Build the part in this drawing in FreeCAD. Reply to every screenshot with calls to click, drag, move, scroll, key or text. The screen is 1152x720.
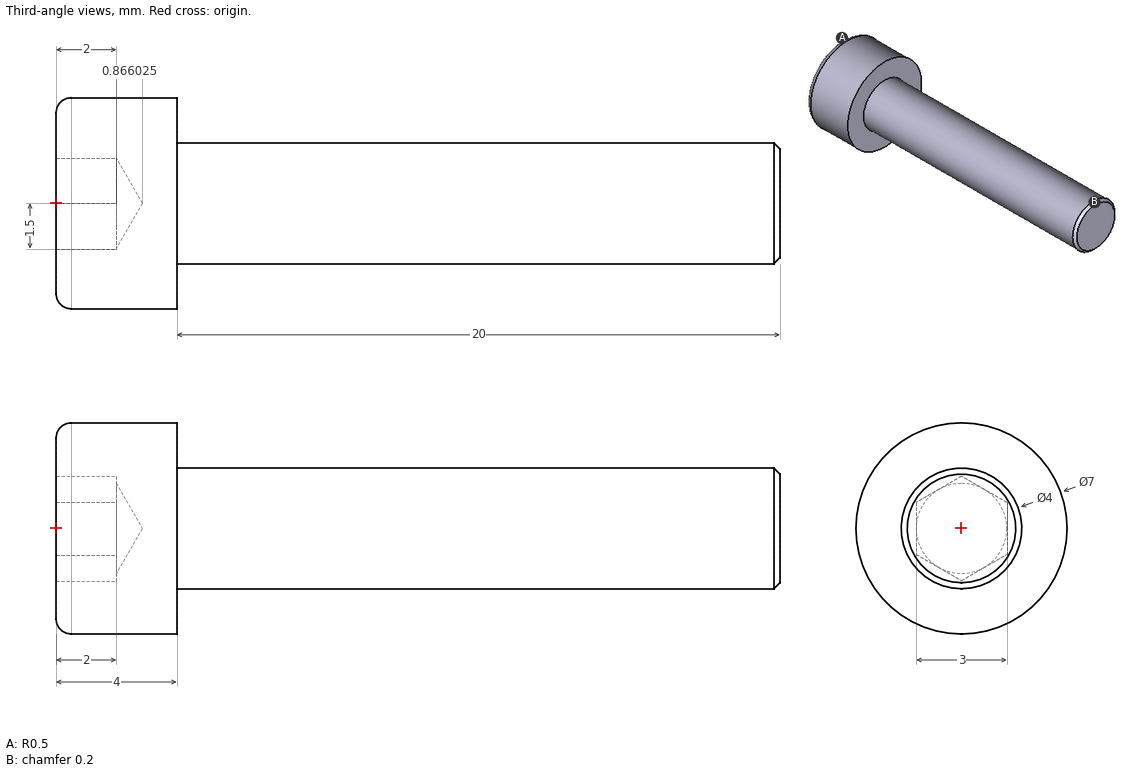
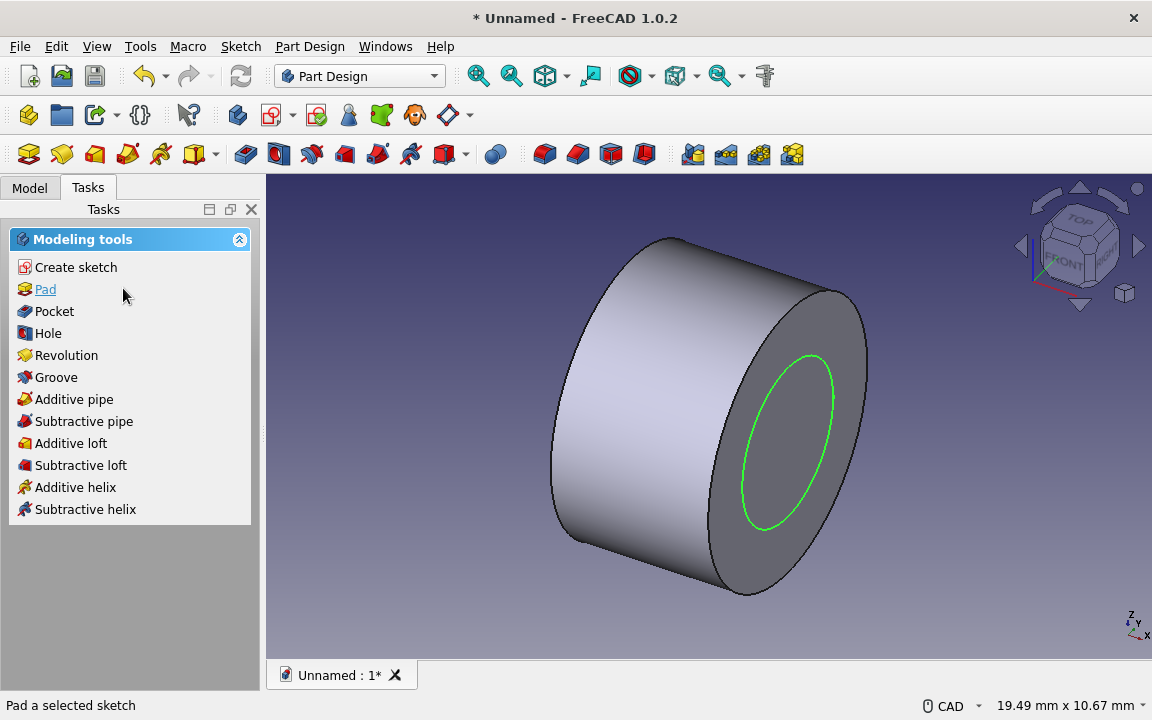
click(29, 154)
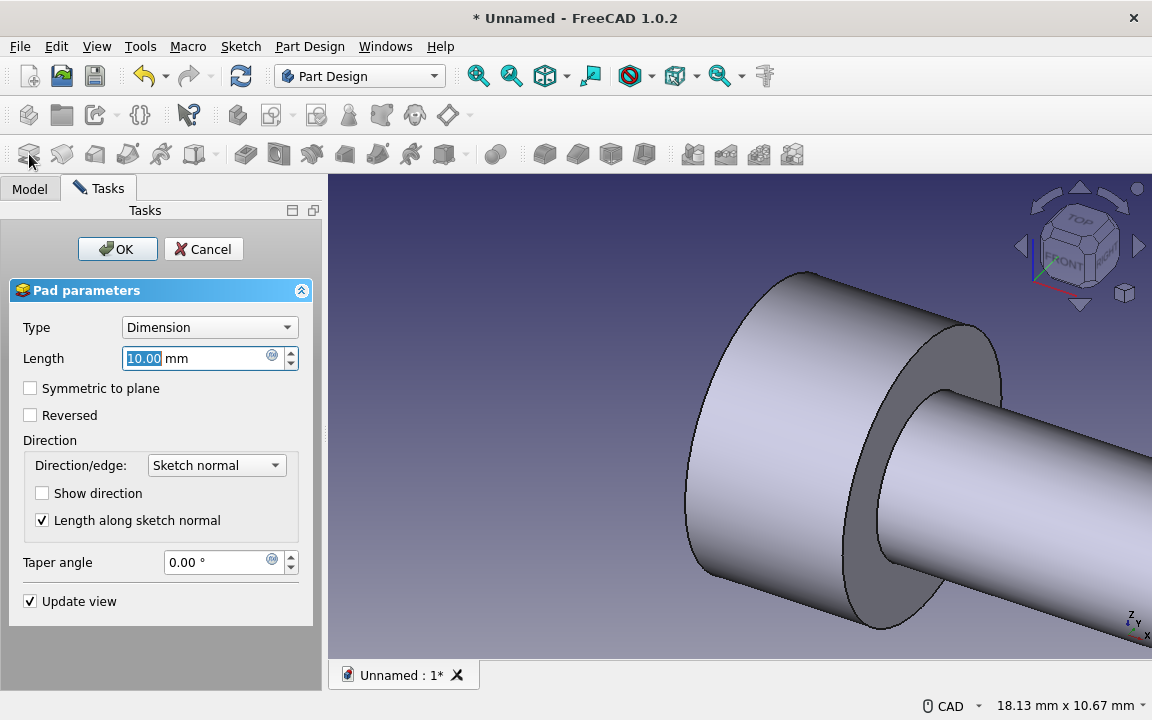
text(20)
key(Tab)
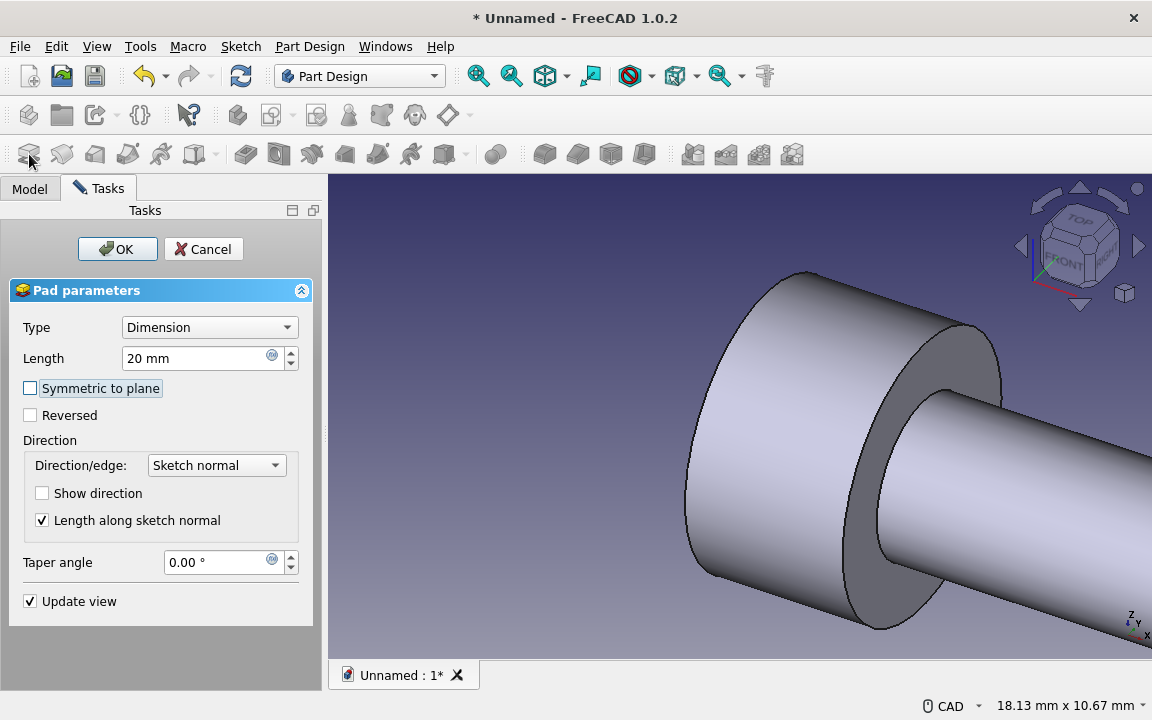
click(118, 249)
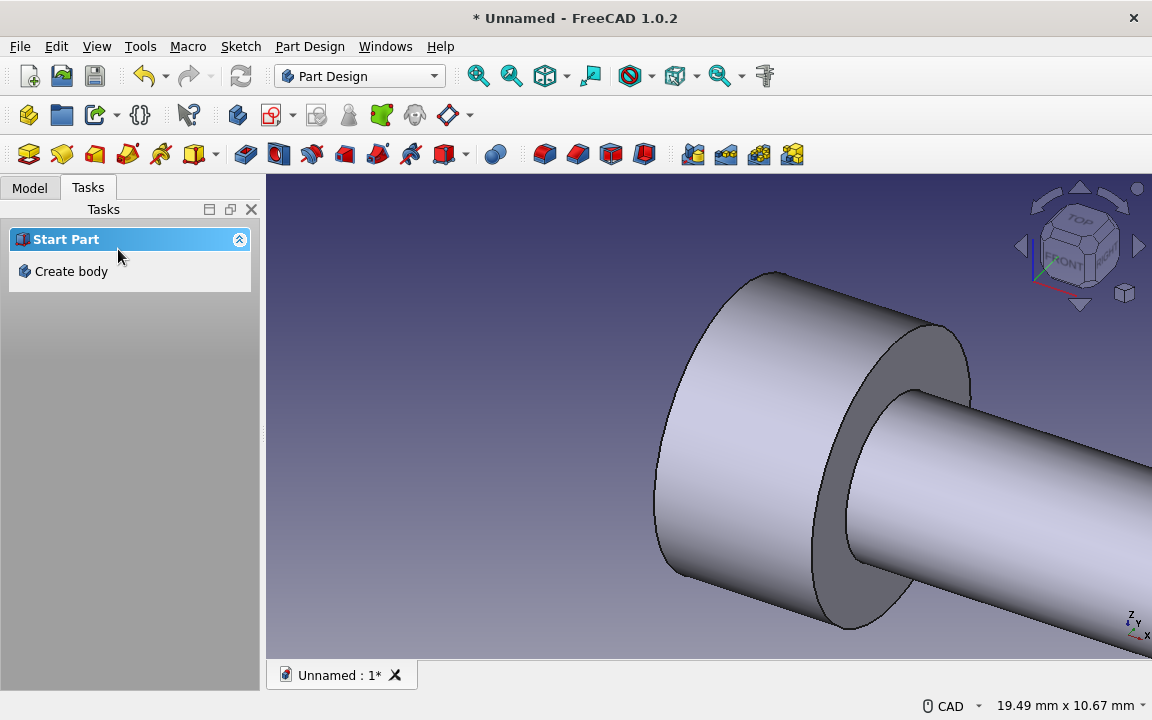
click(479, 76)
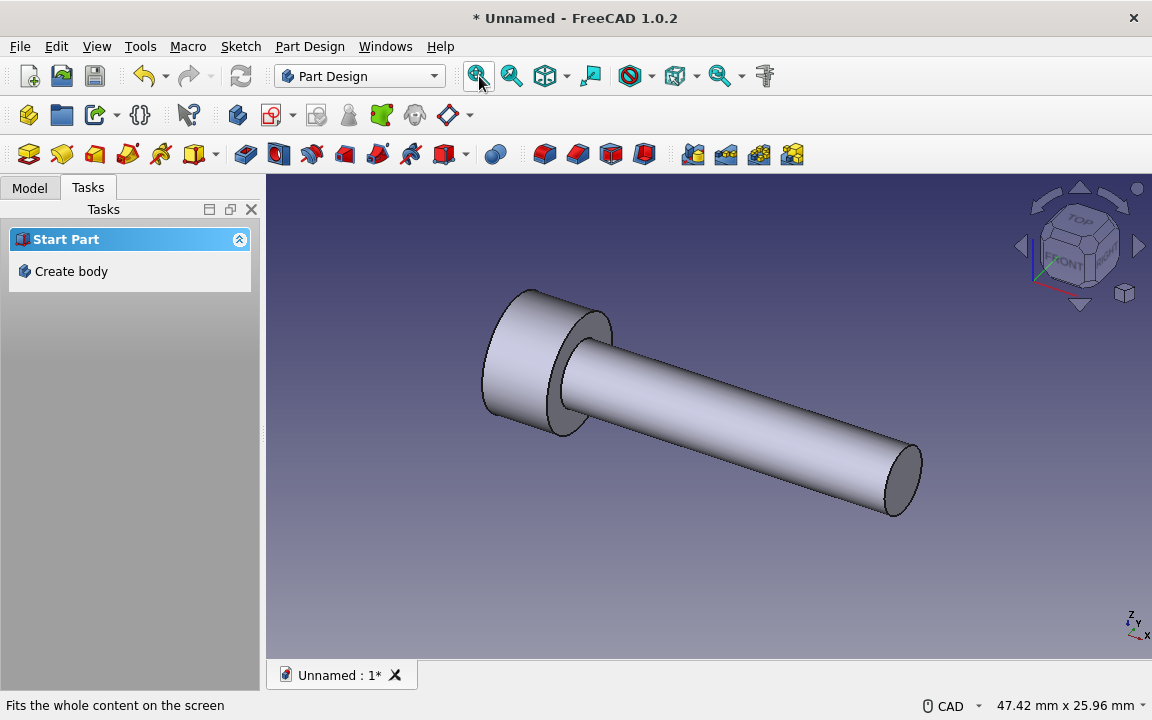
key(6)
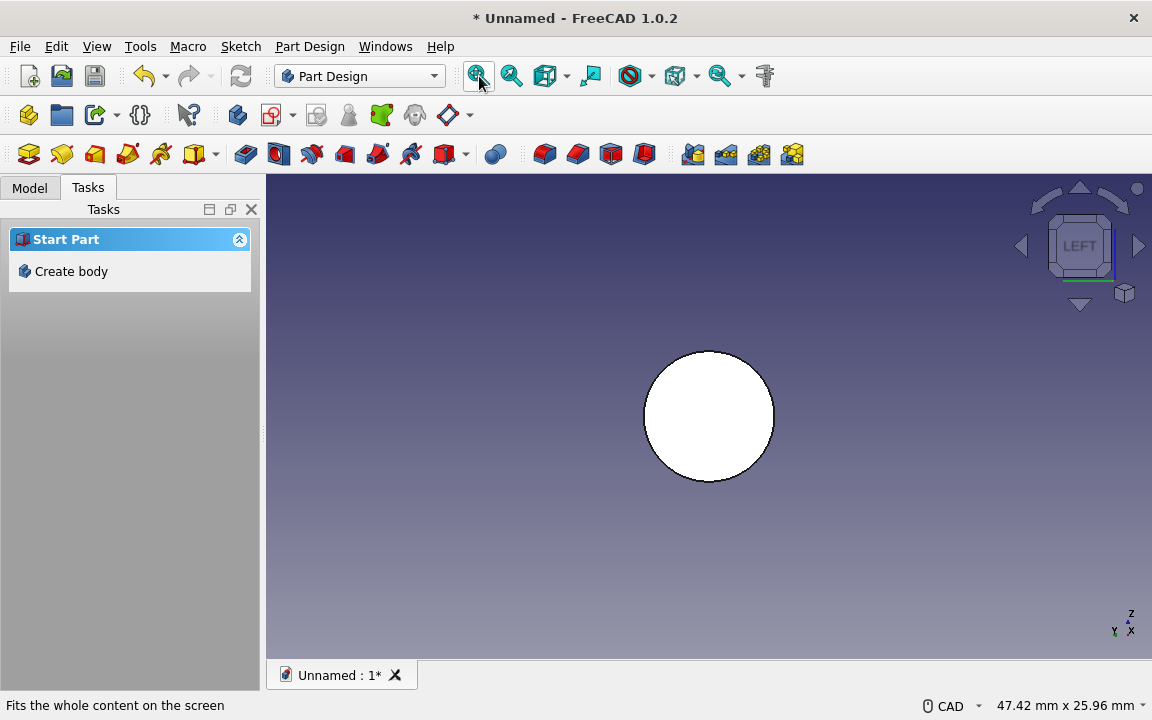
click(479, 76)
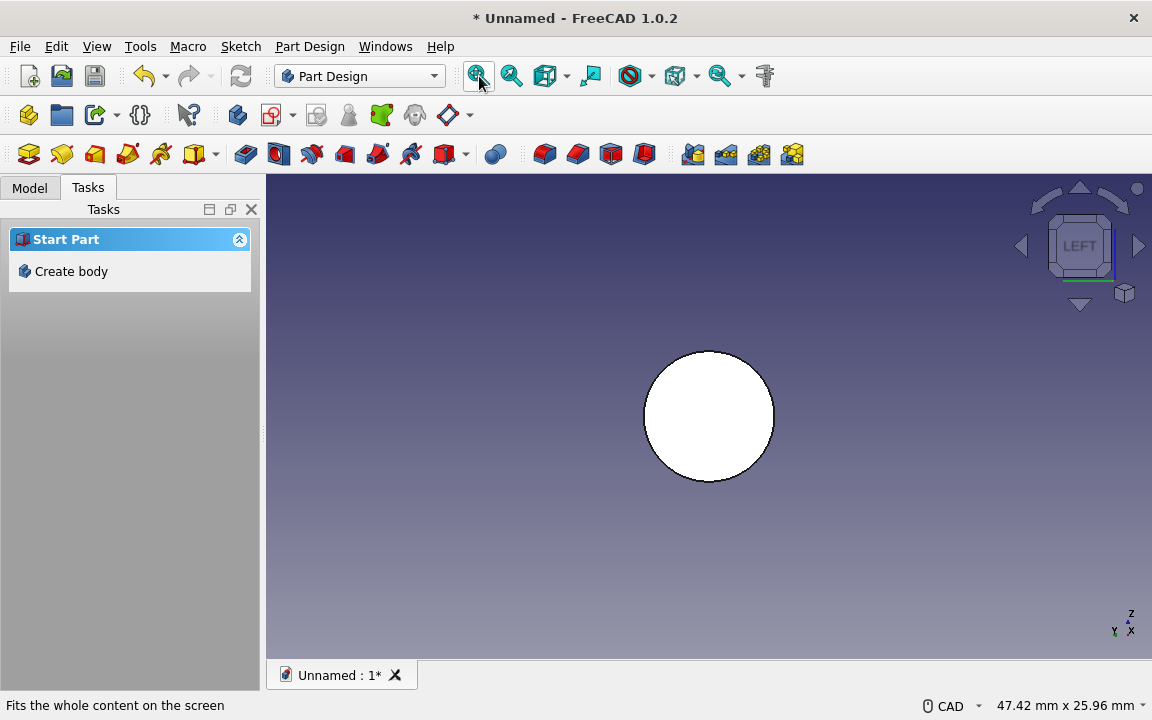
click(709, 415)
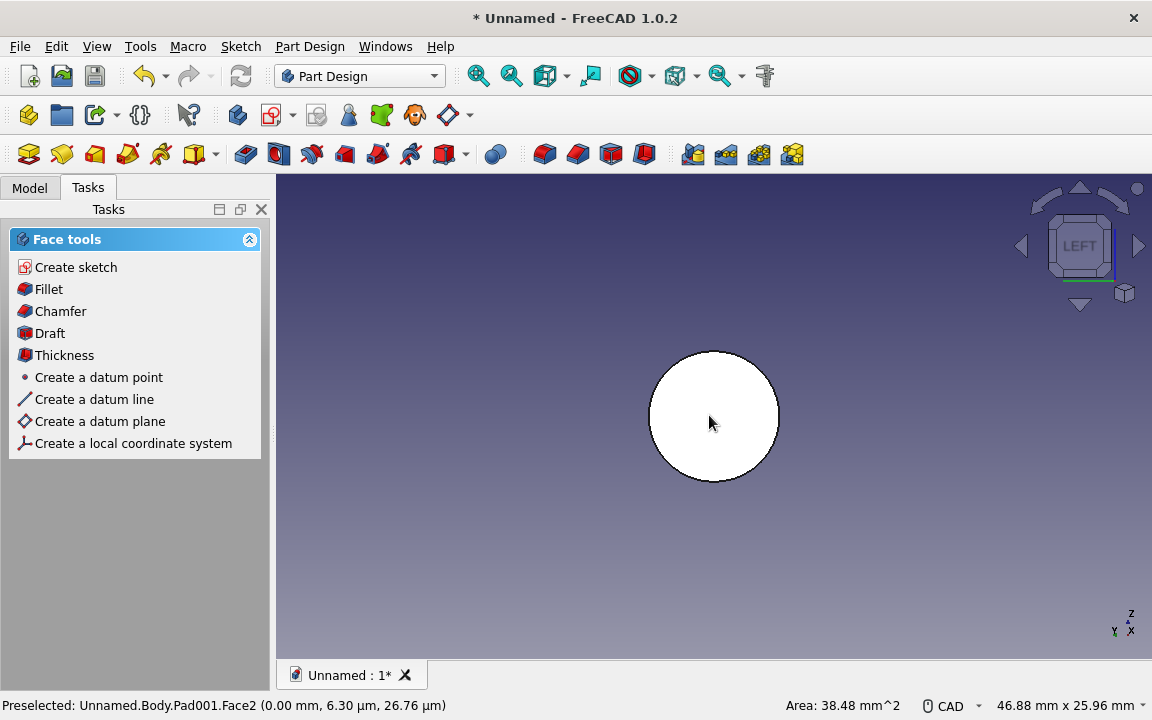
click(270, 116)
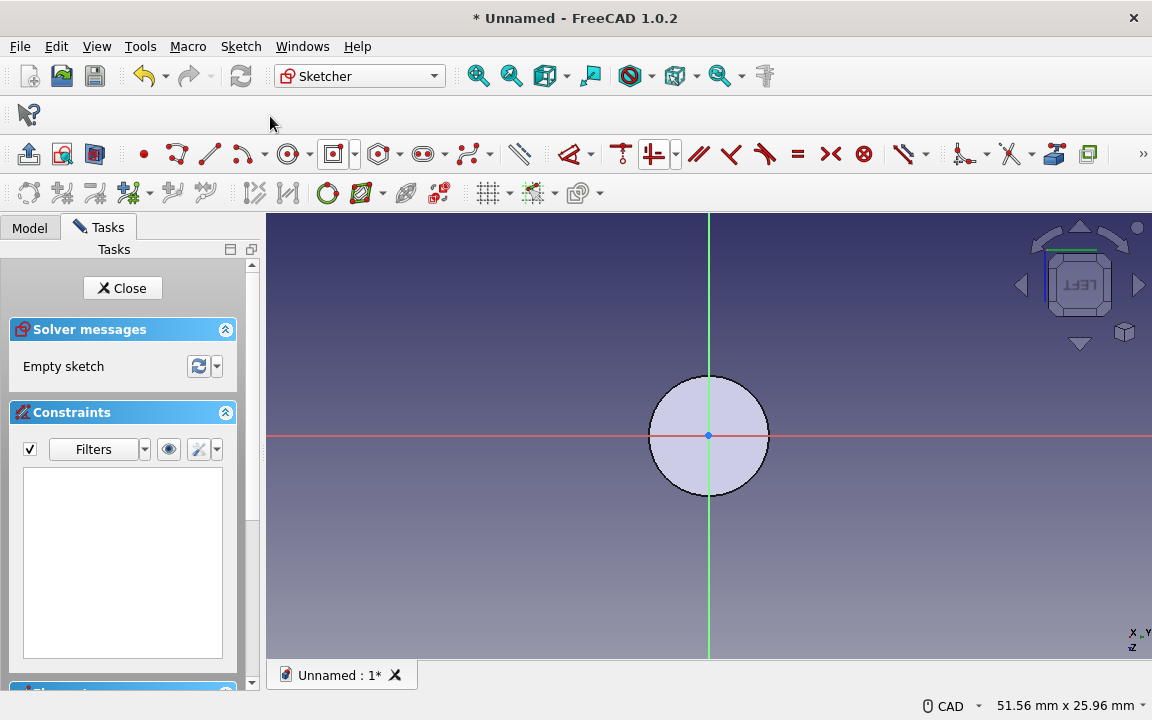
scroll(726, 436, up, 8)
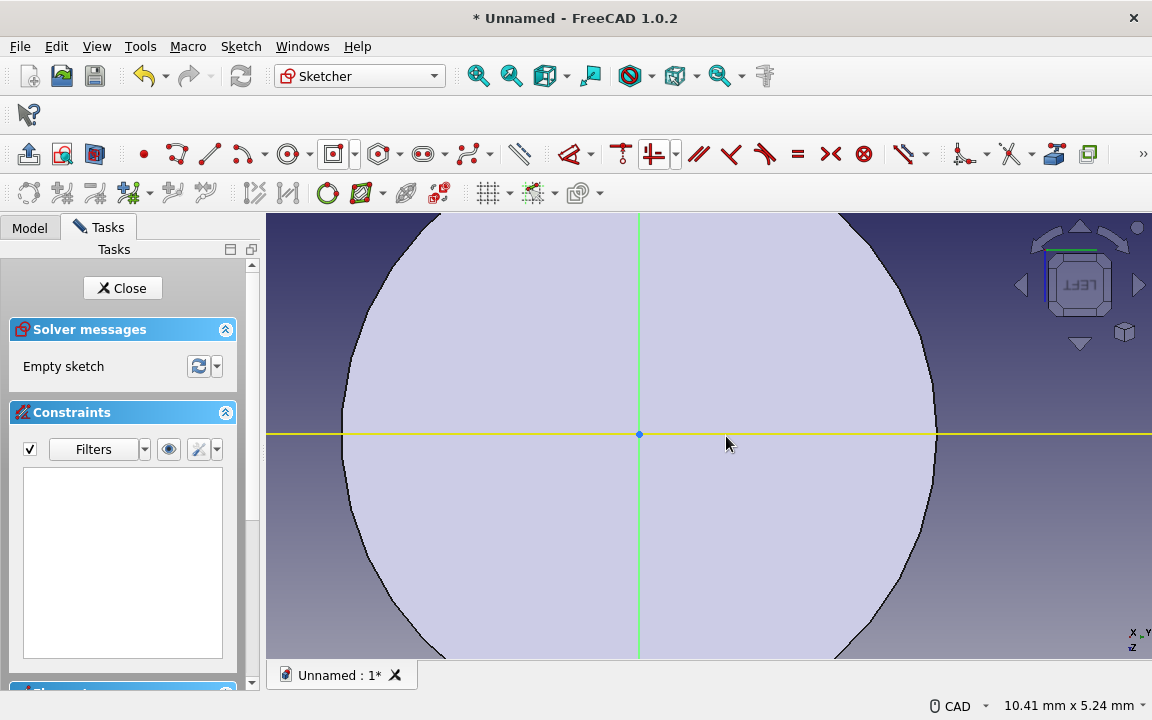
click(378, 154)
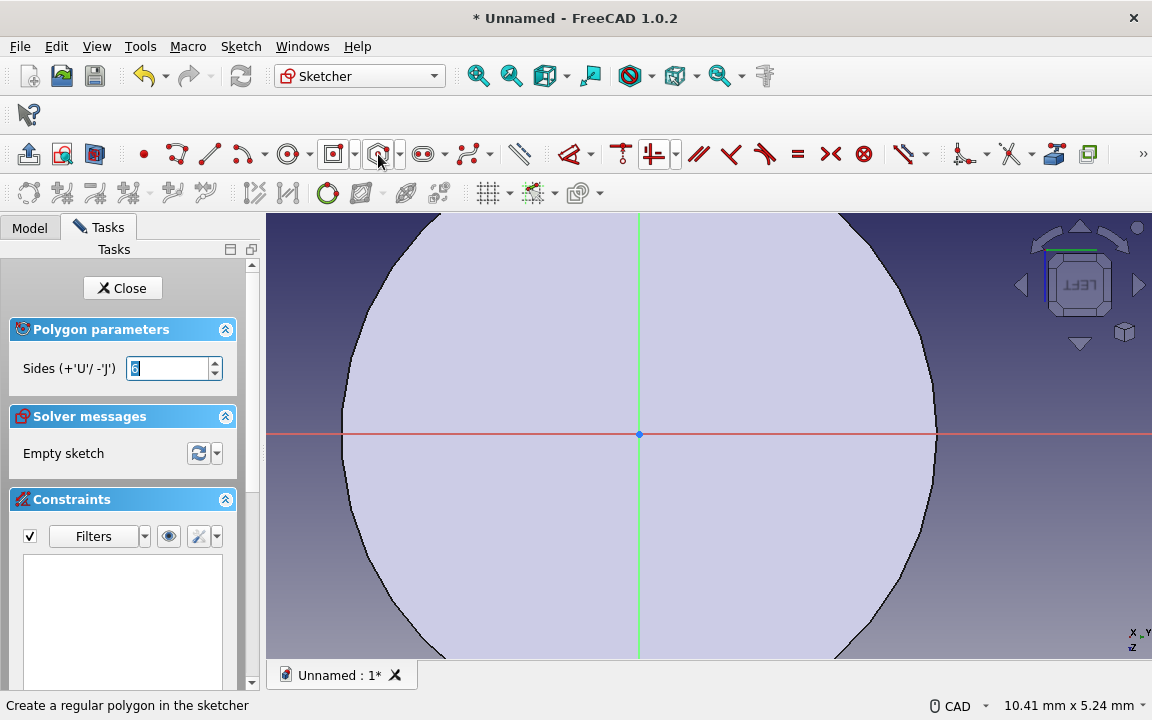
click(639, 434)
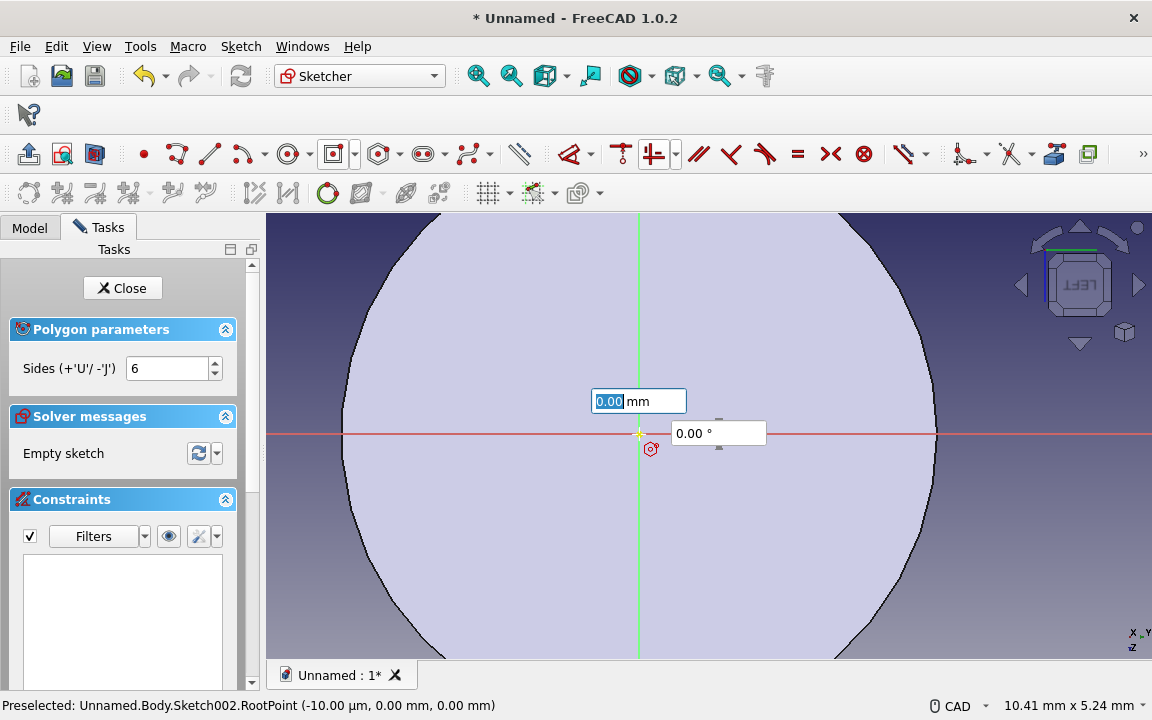
click(639, 287)
right_click(639, 287)